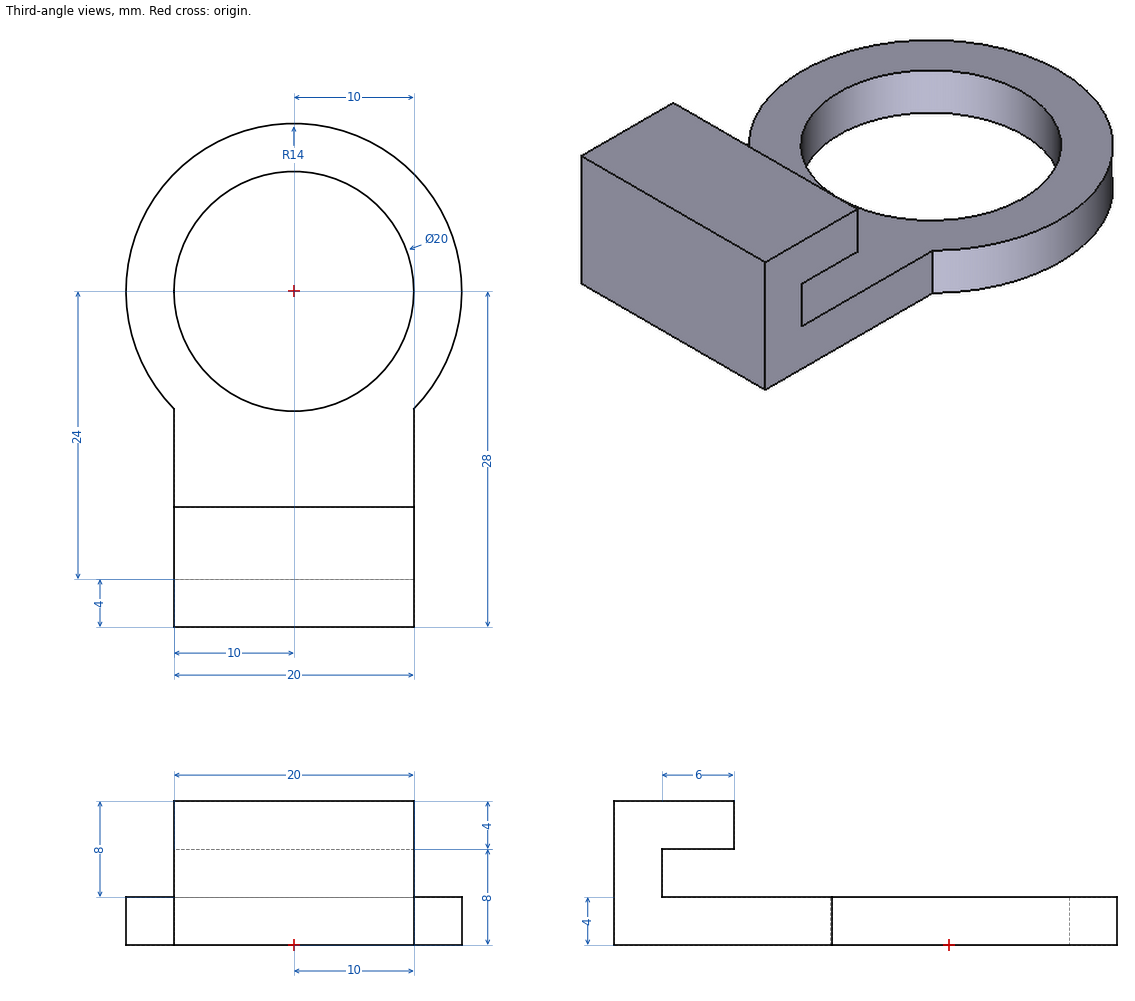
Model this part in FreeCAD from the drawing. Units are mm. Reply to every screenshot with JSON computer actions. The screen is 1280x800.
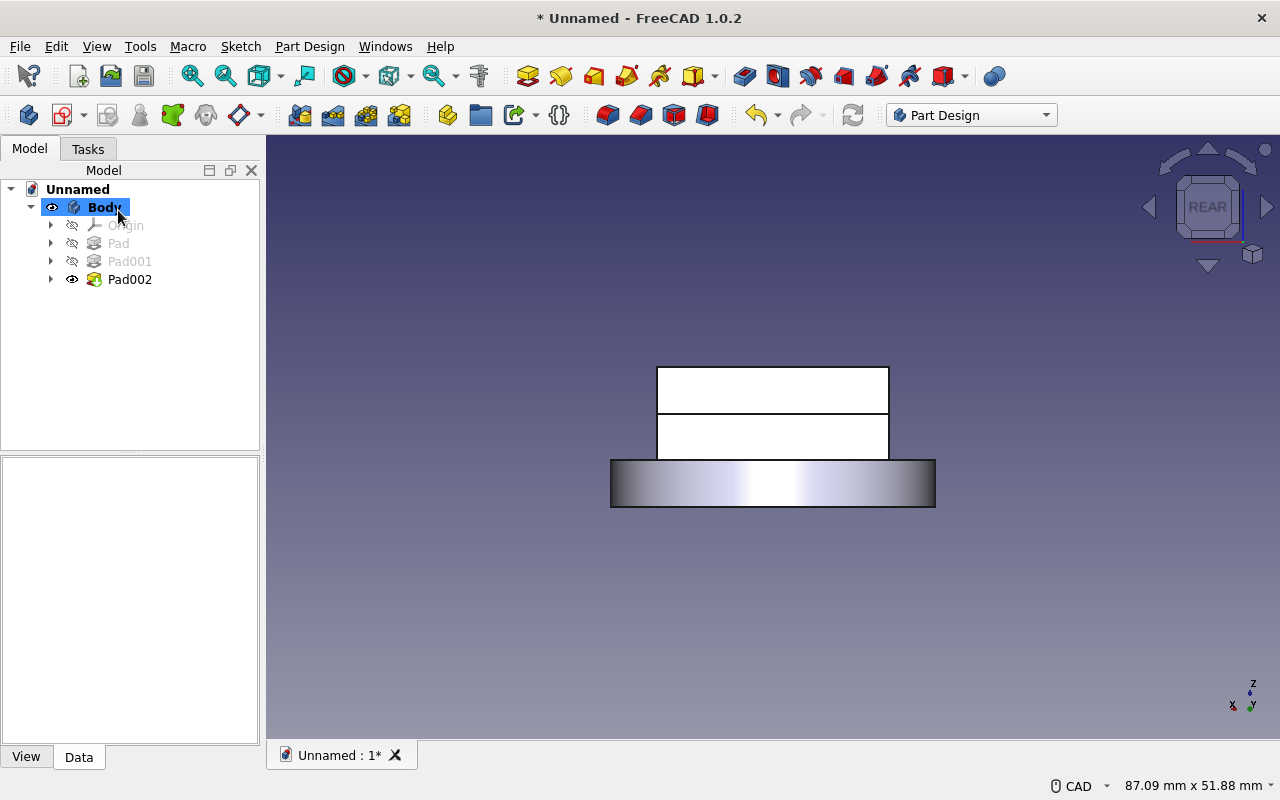
{"action": "left_click", "coordinate": [193, 76]}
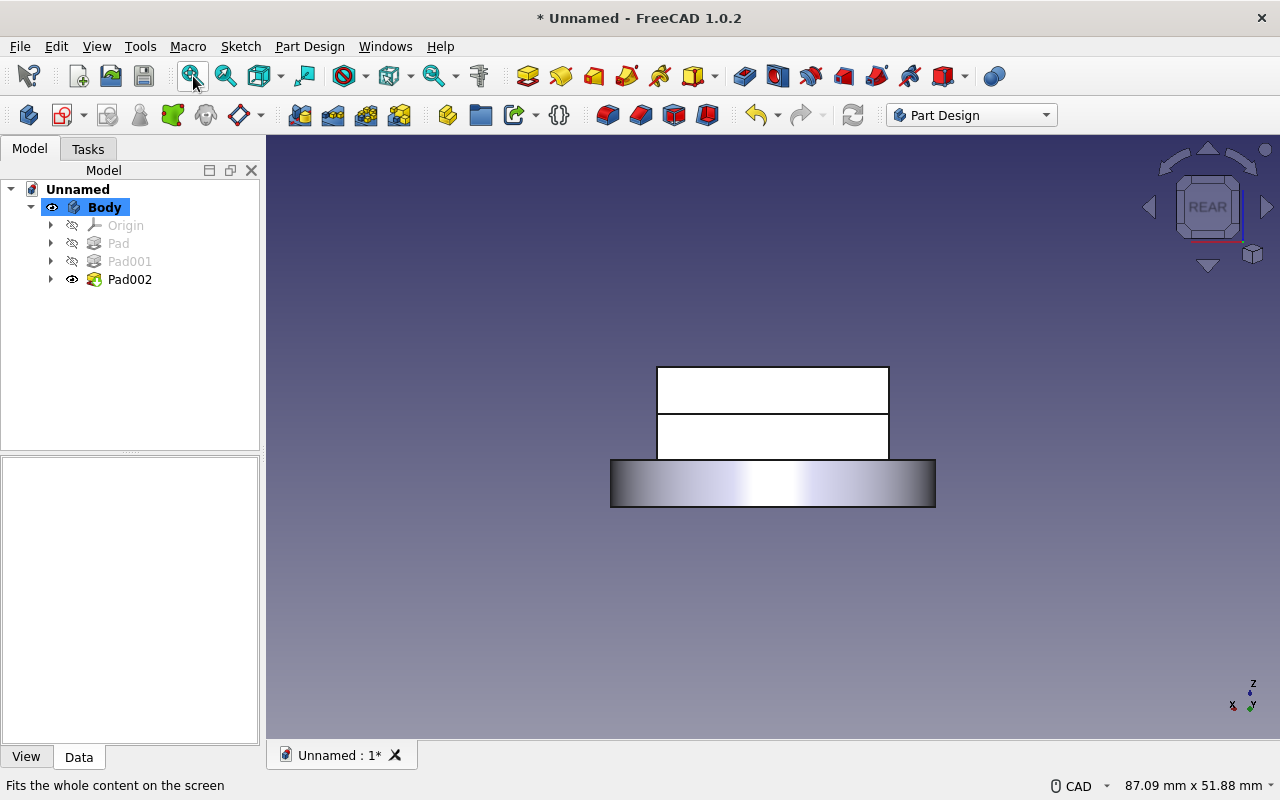
{"action": "key", "text": "0"}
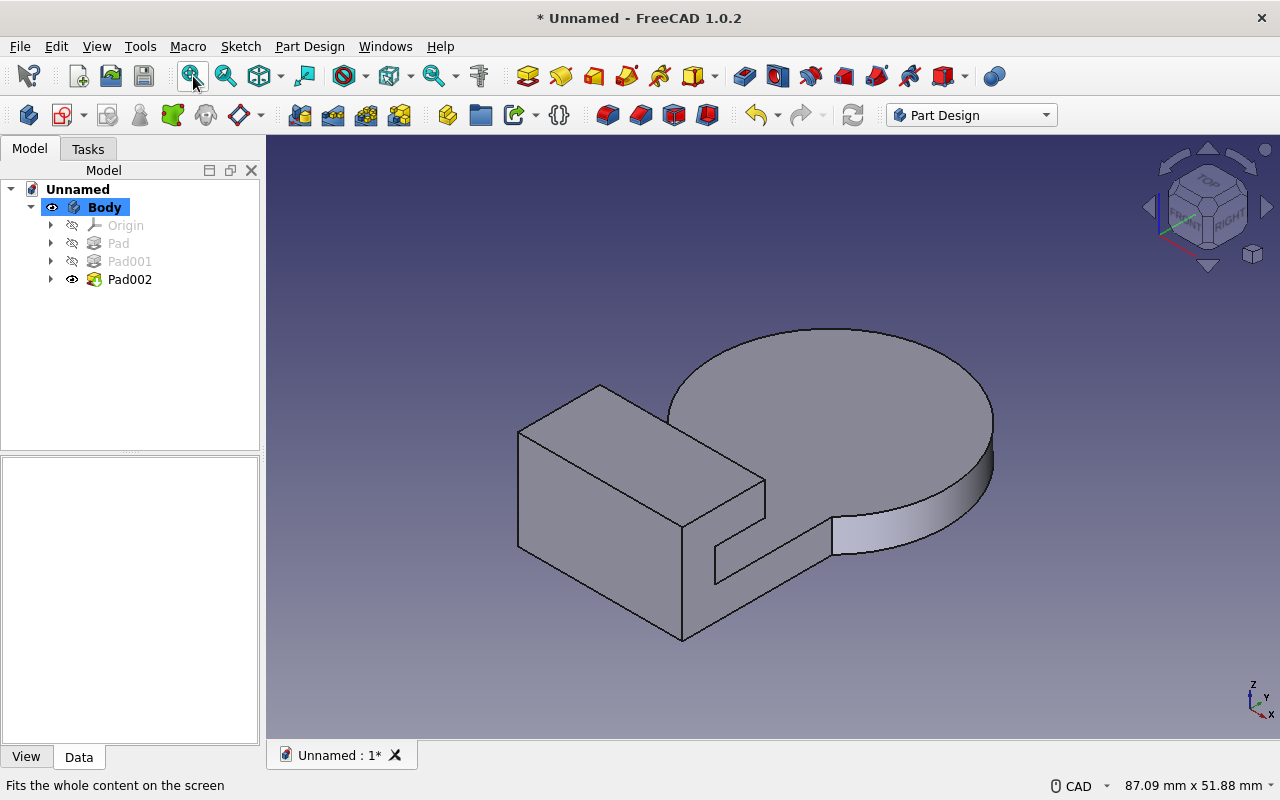
{"action": "left_click", "coordinate": [834, 420]}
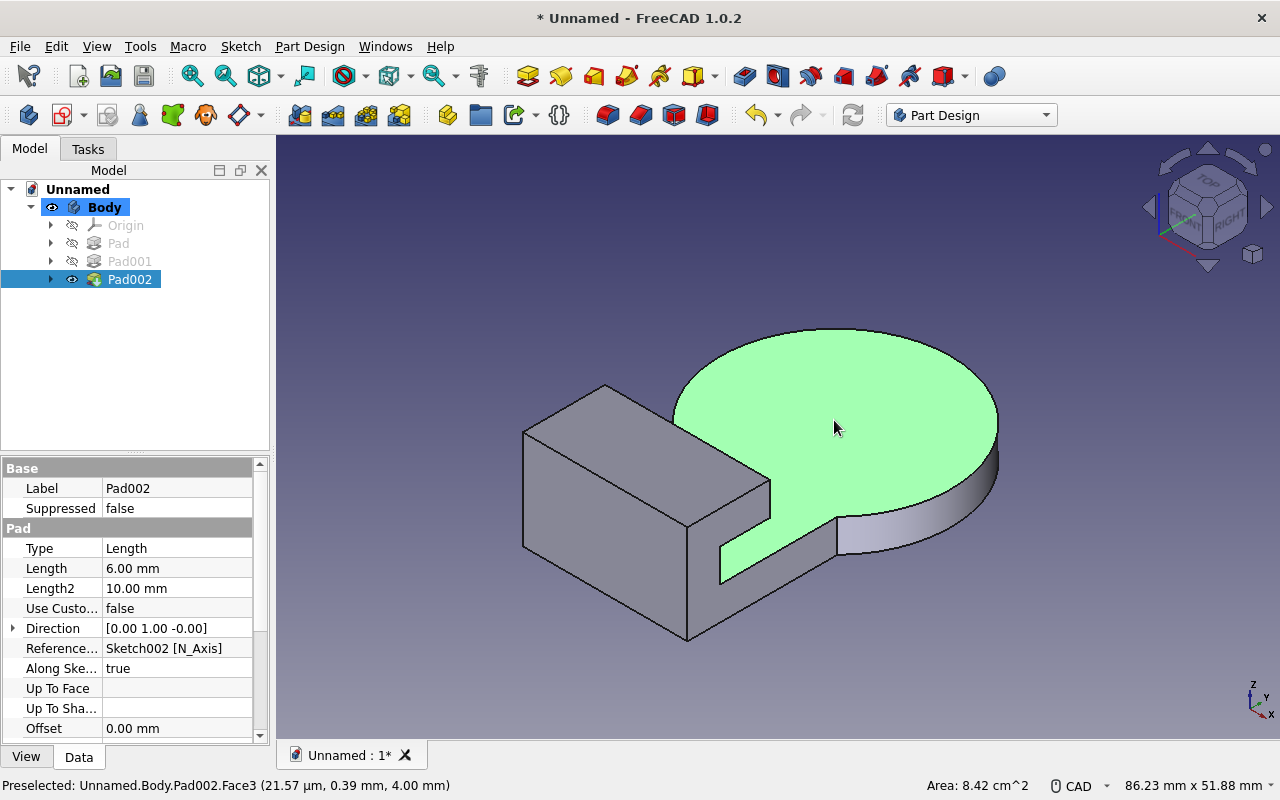
{"action": "left_click", "coordinate": [62, 116]}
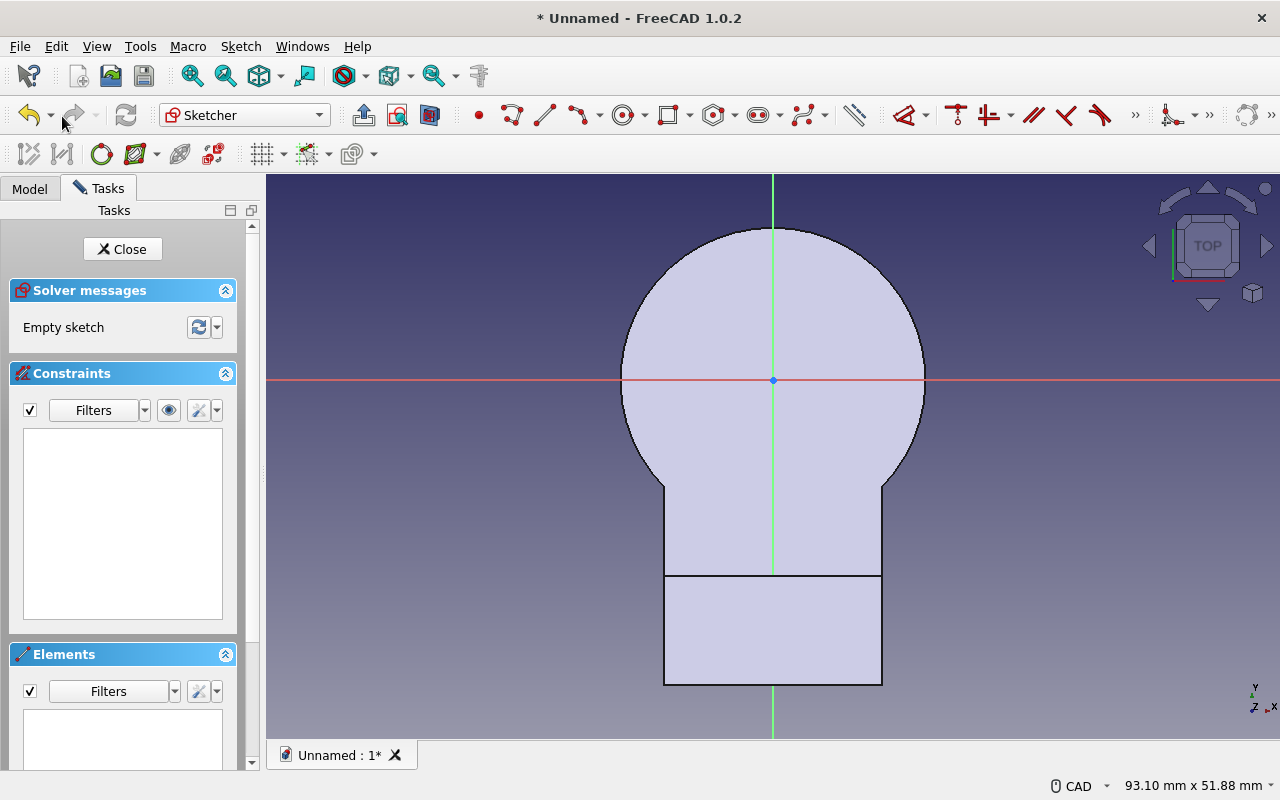
{"action": "key", "text": "q s"}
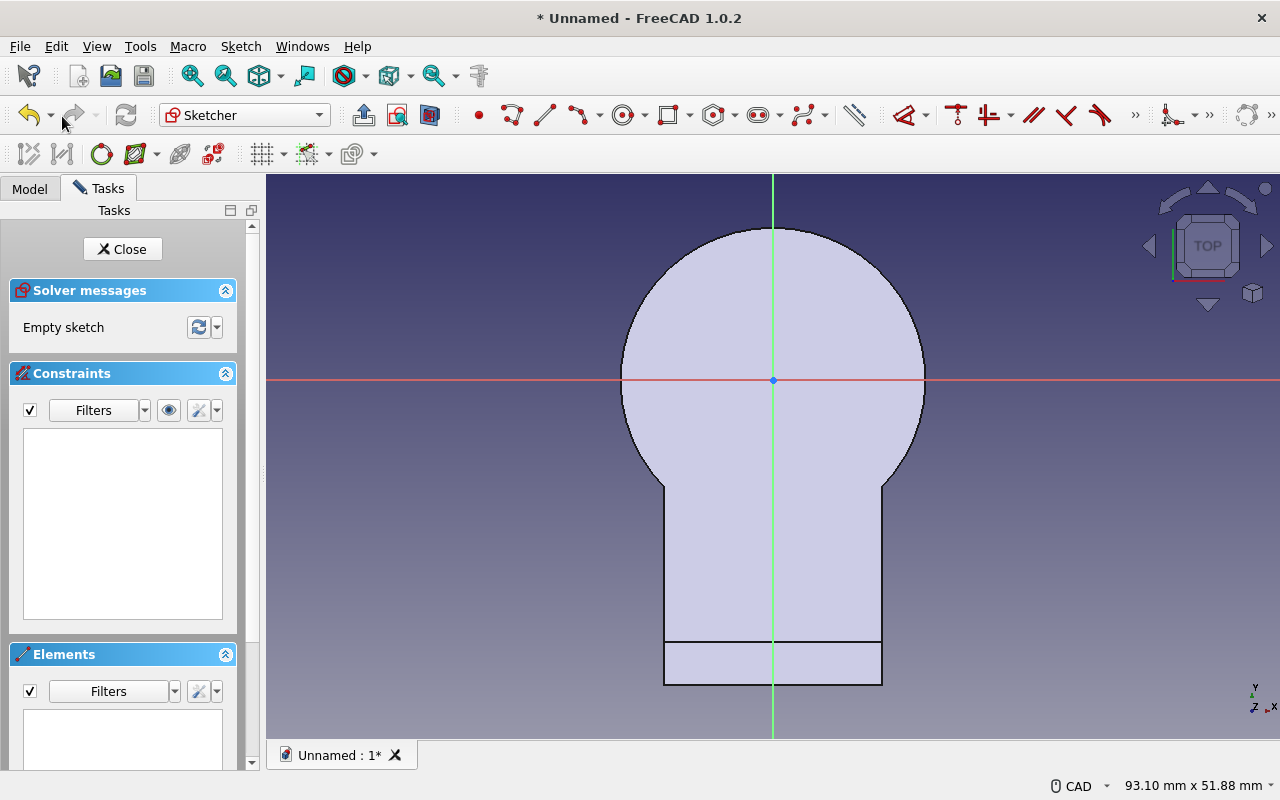
{"action": "scroll", "coordinate": [856, 288], "scroll_direction": "up", "scroll_amount": 3}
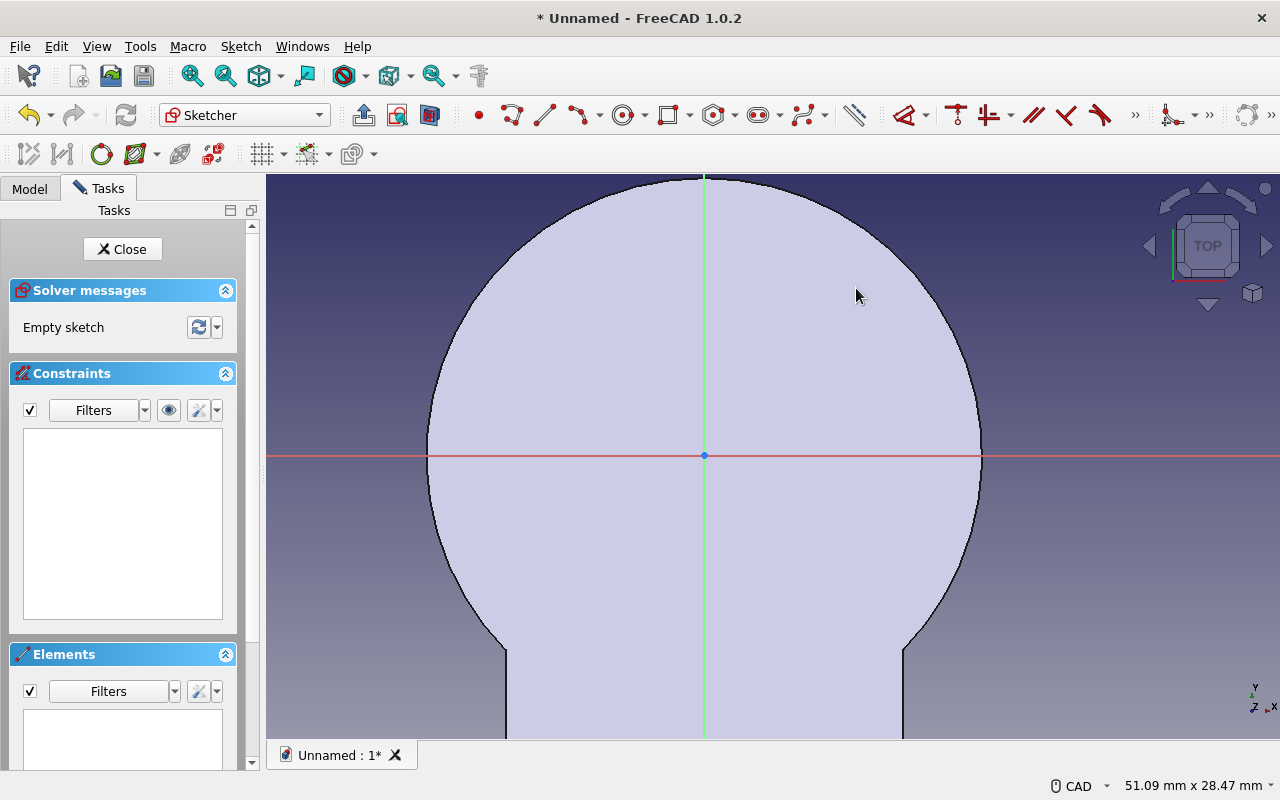
{"action": "left_click", "coordinate": [622, 116]}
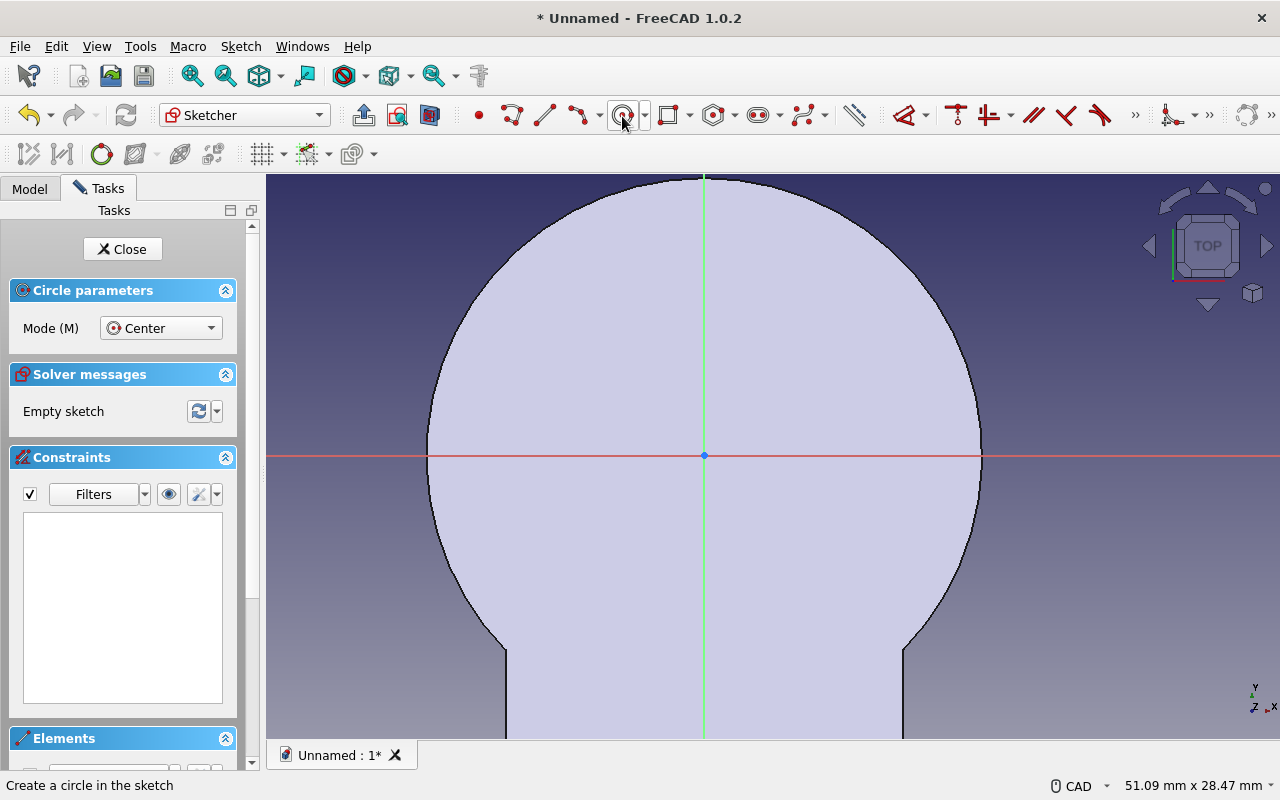
{"action": "left_click", "coordinate": [704, 456]}
{"action": "left_click", "coordinate": [845, 316]}
{"action": "key", "text": "Escape"}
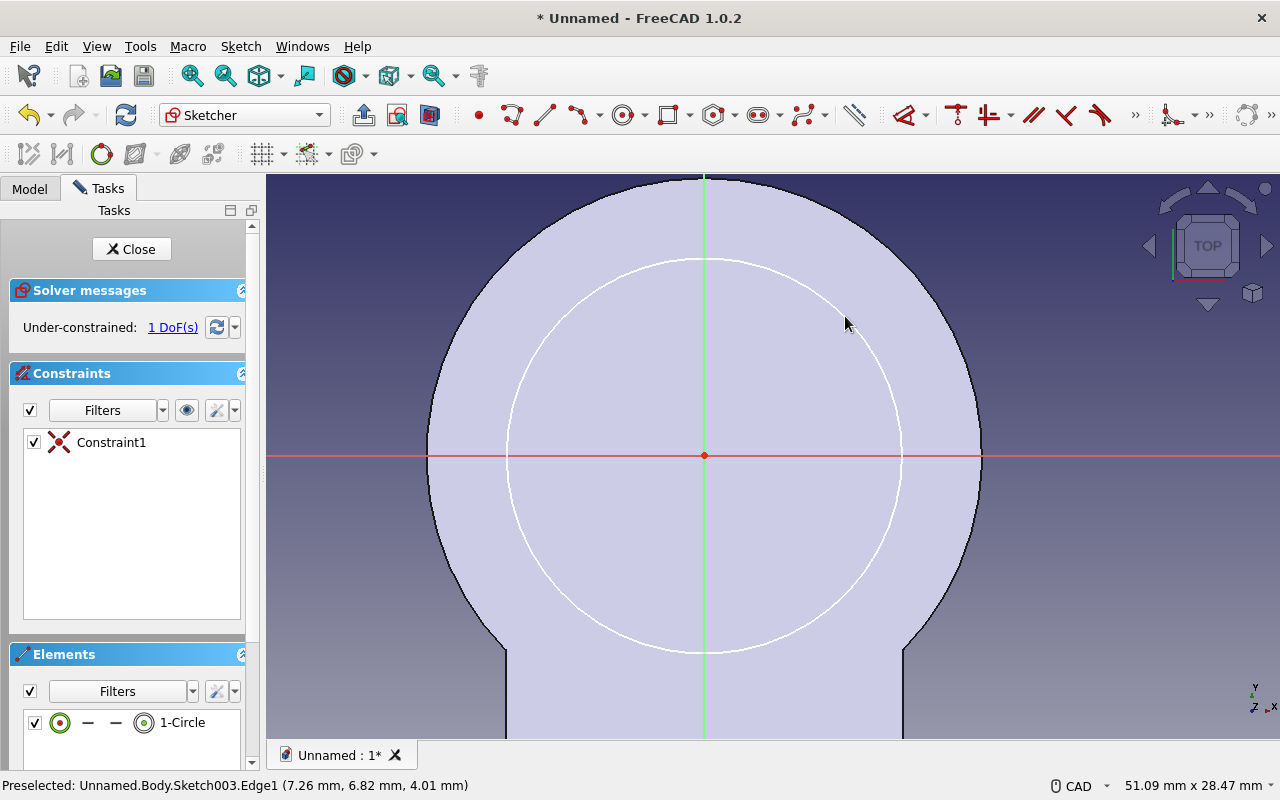
{"action": "key", "text": "d"}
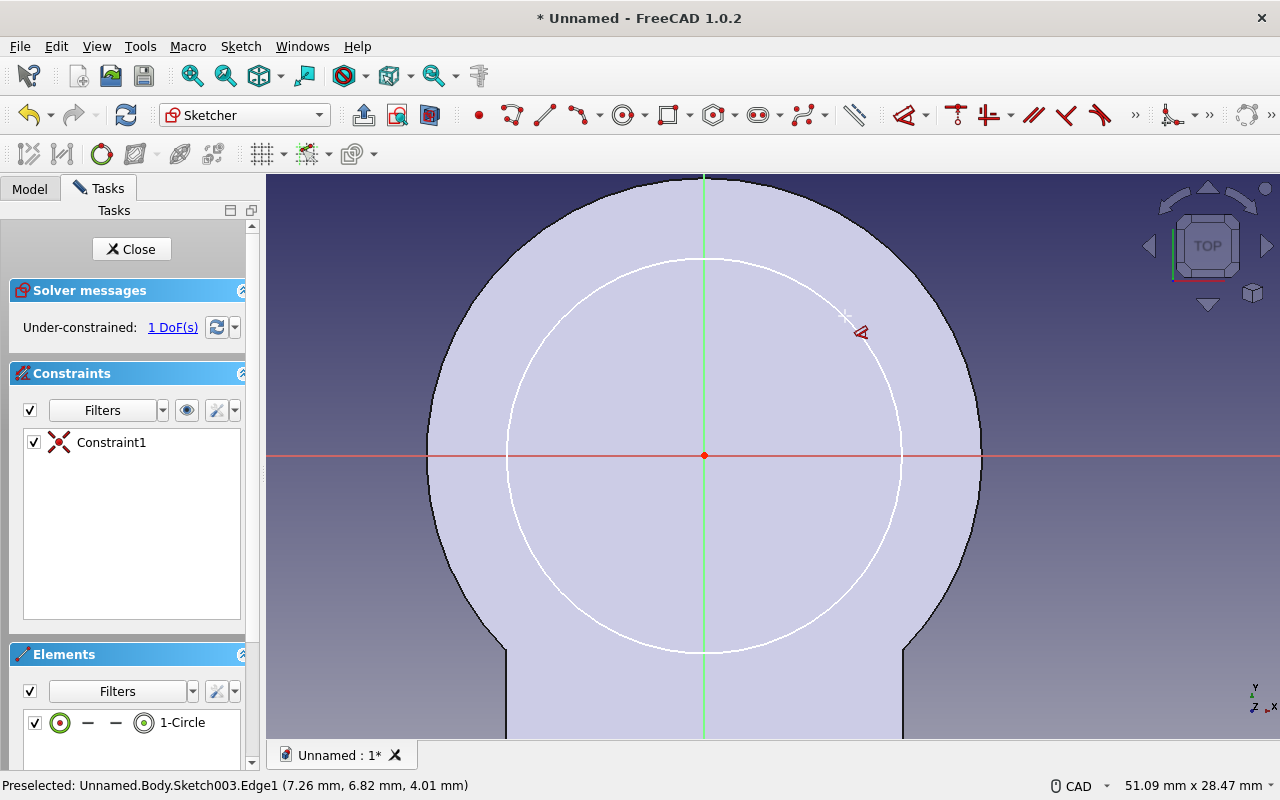
{"action": "left_click", "coordinate": [844, 316]}
{"action": "left_click", "coordinate": [867, 293]}